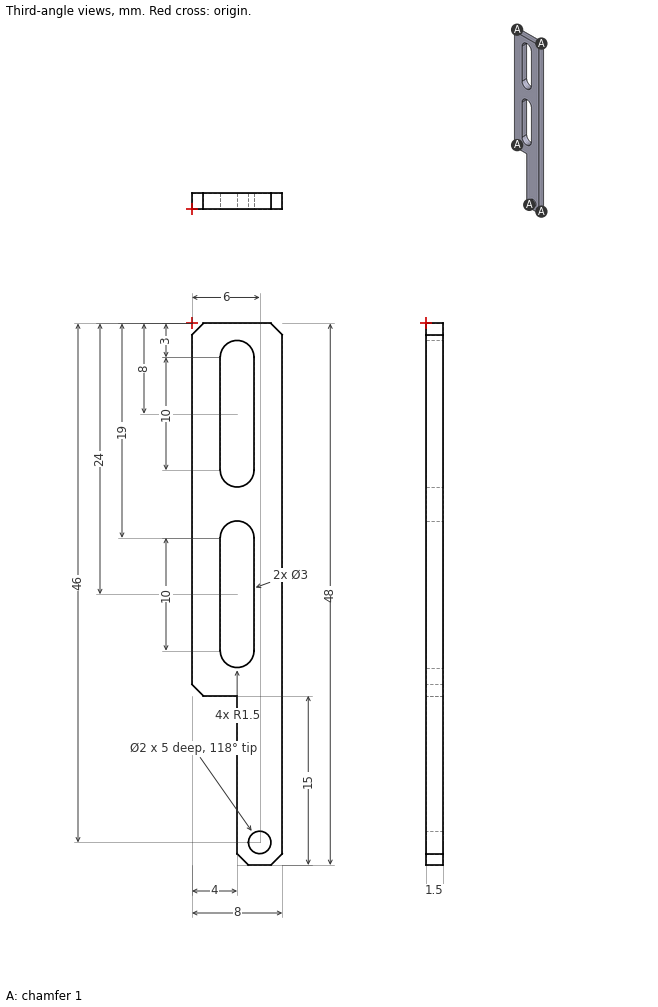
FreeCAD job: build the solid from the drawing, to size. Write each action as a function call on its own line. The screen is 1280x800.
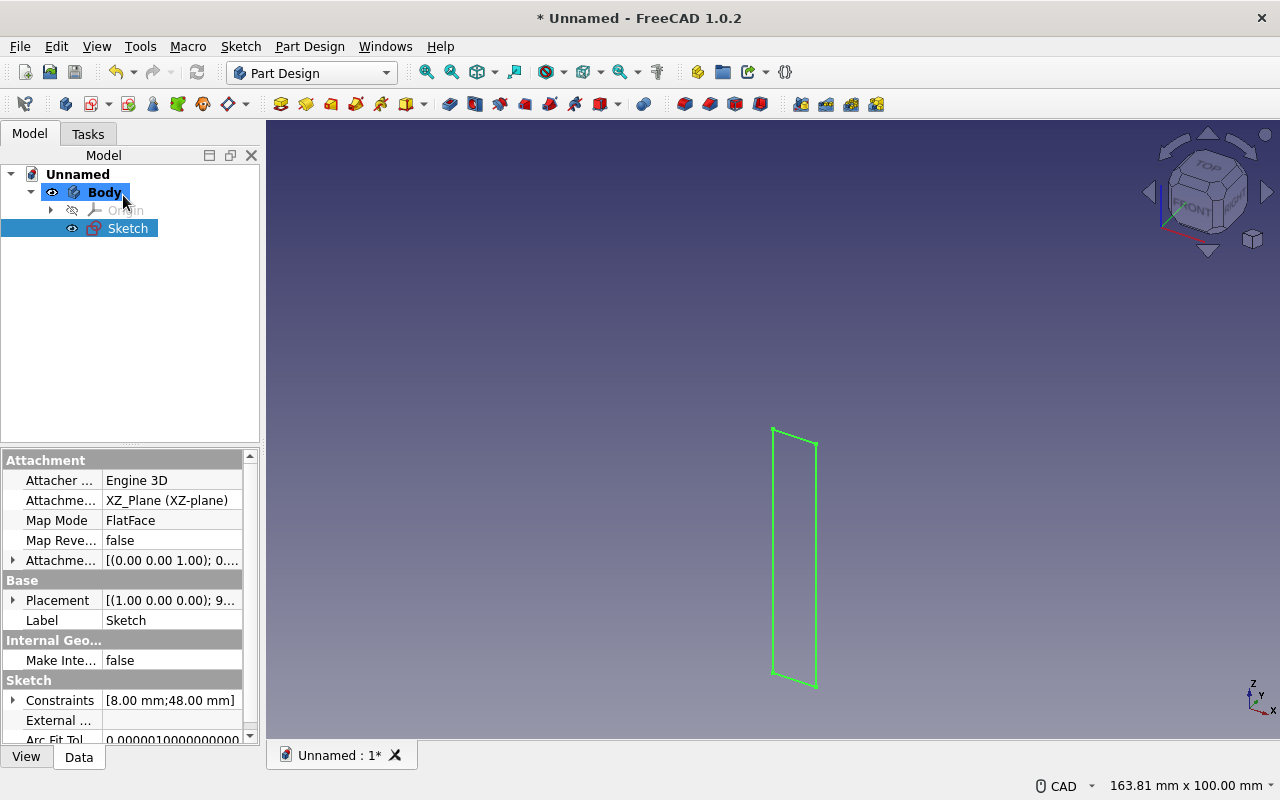
click(281, 104)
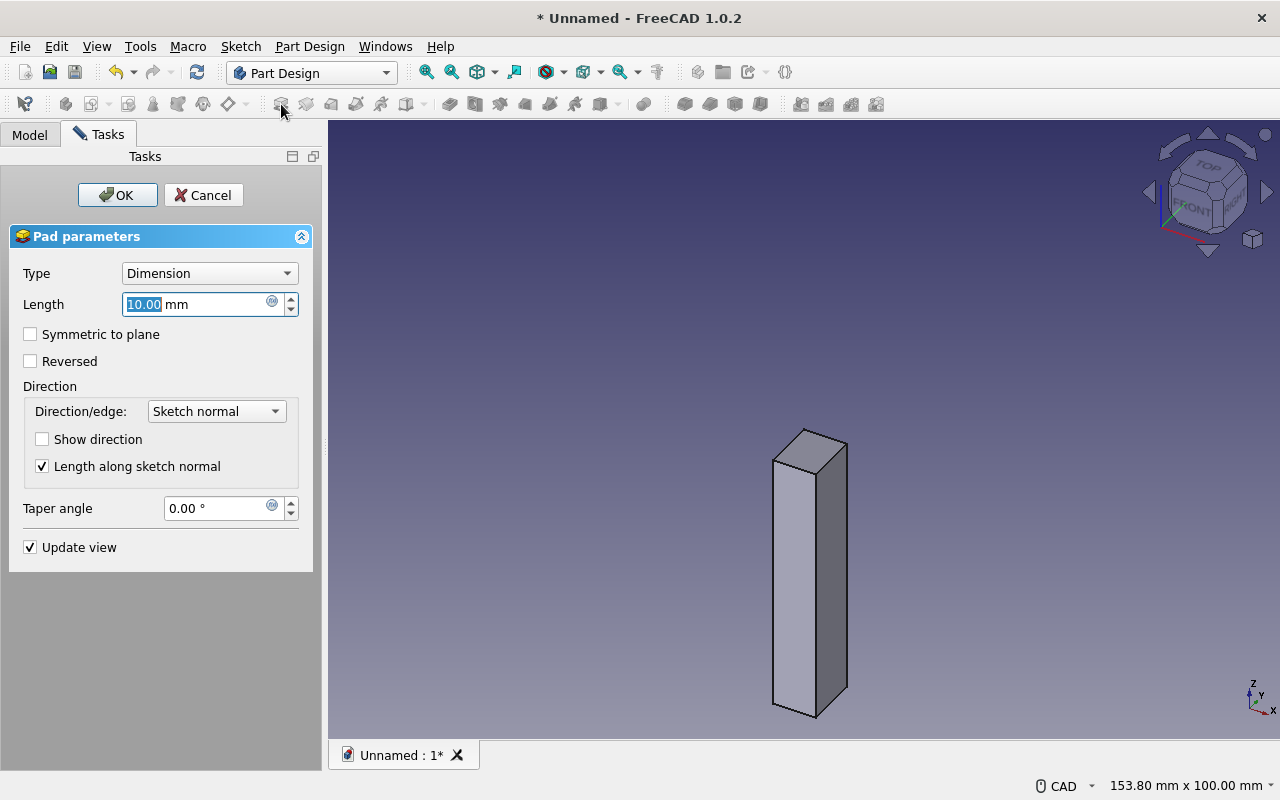
text(1.5)
key(Tab)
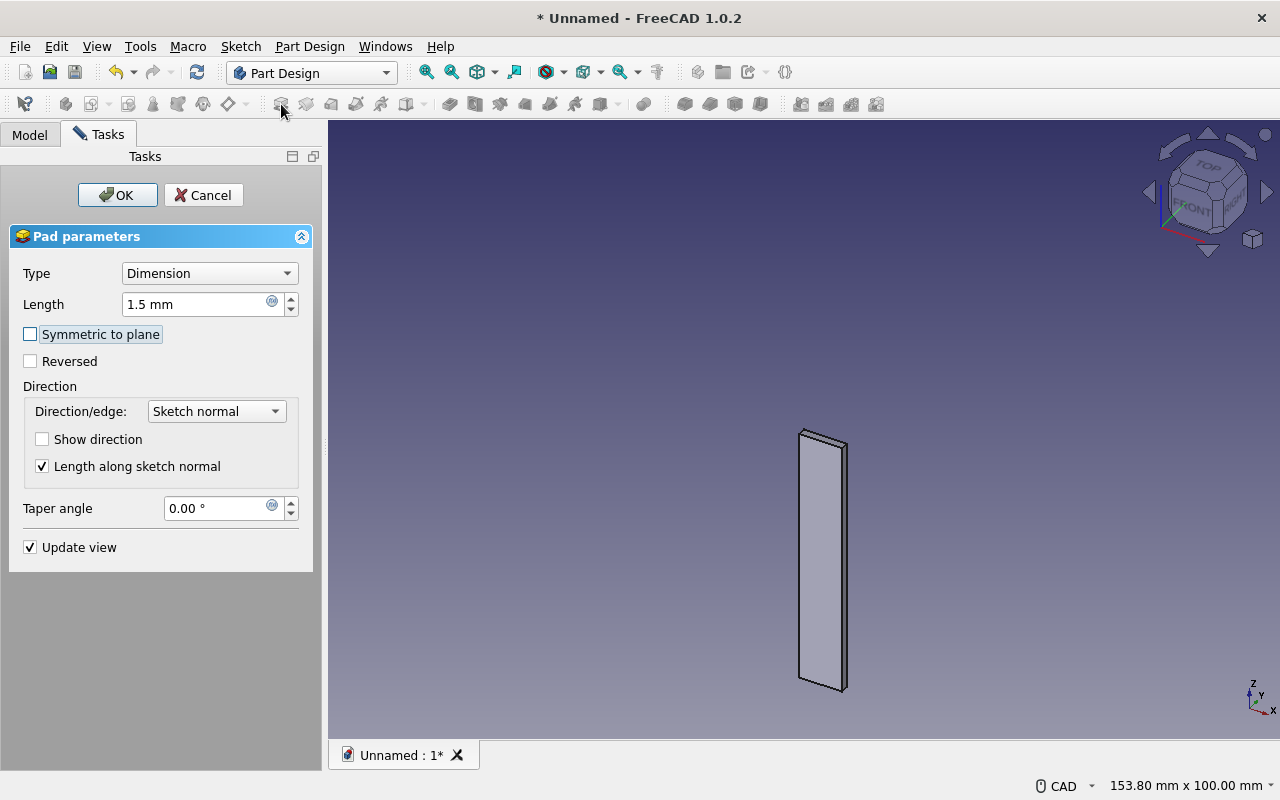
click(31, 361)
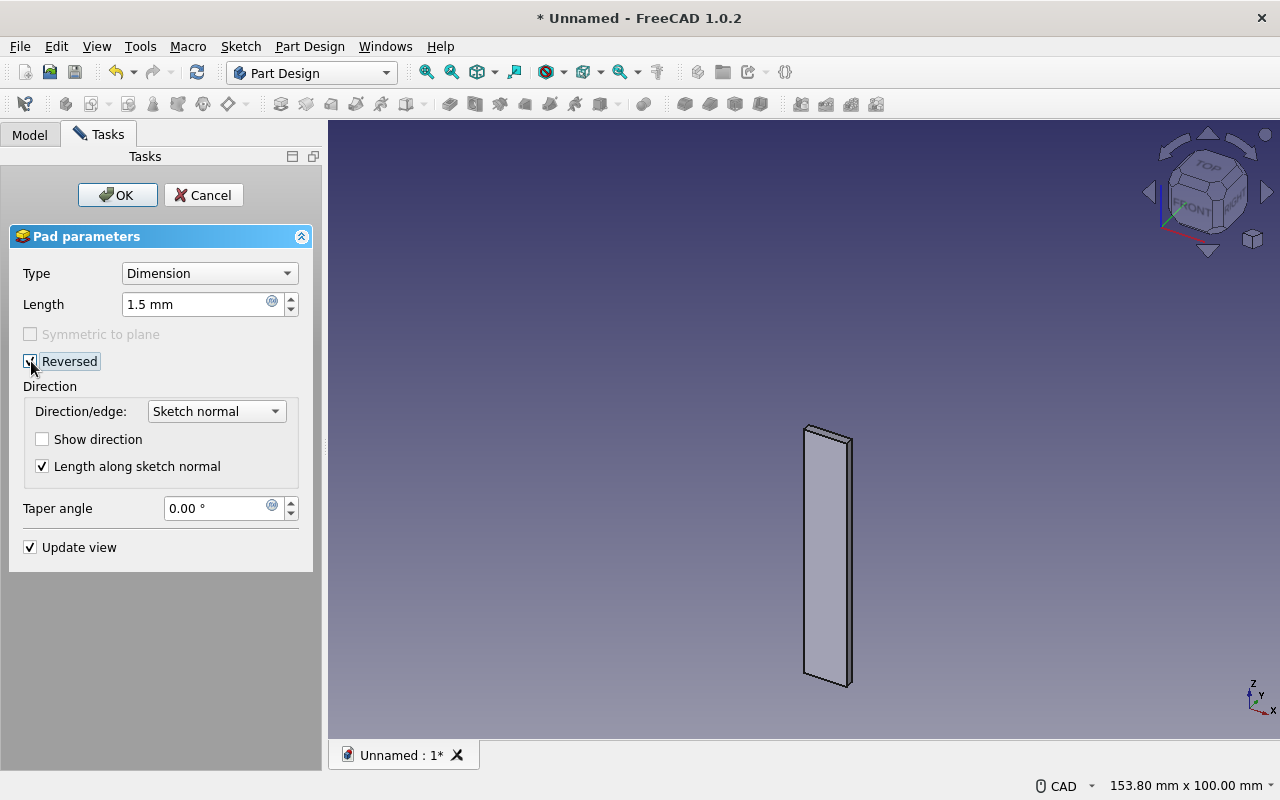
click(118, 195)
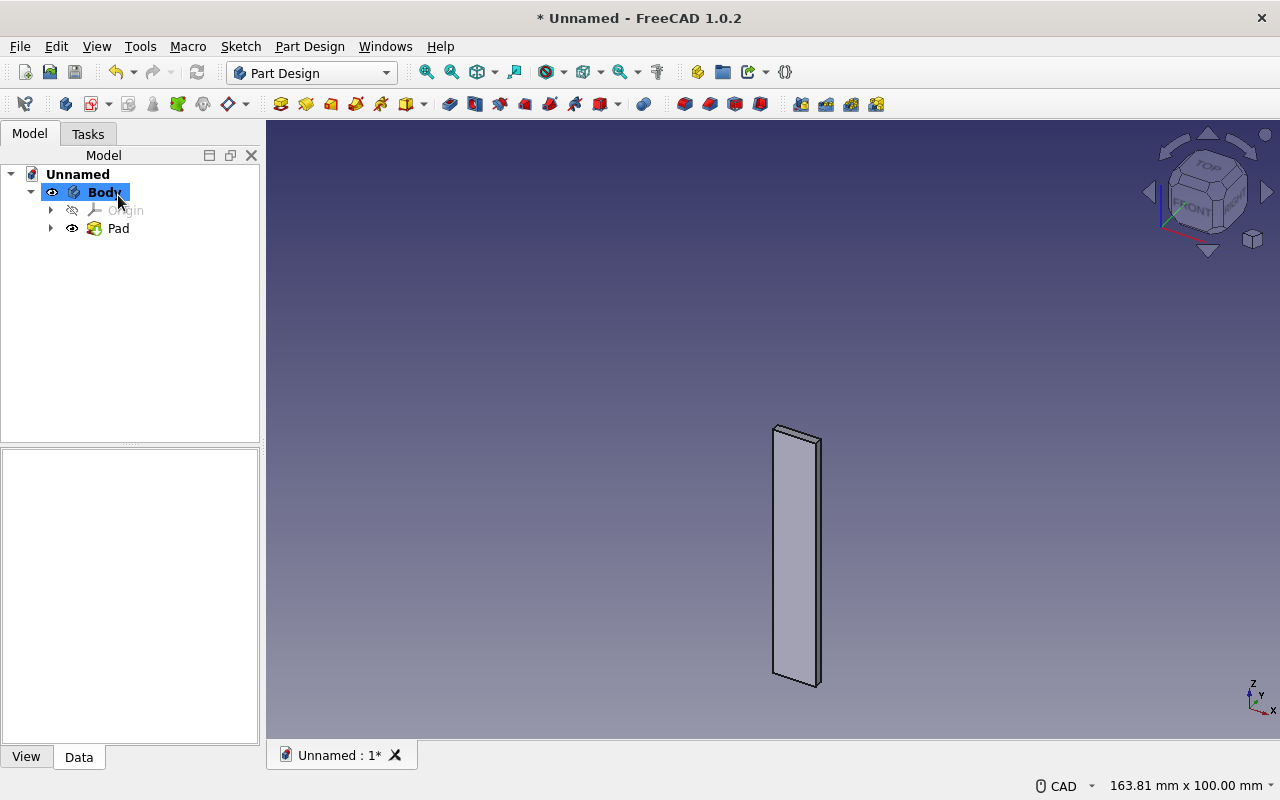
key(v)
key(f)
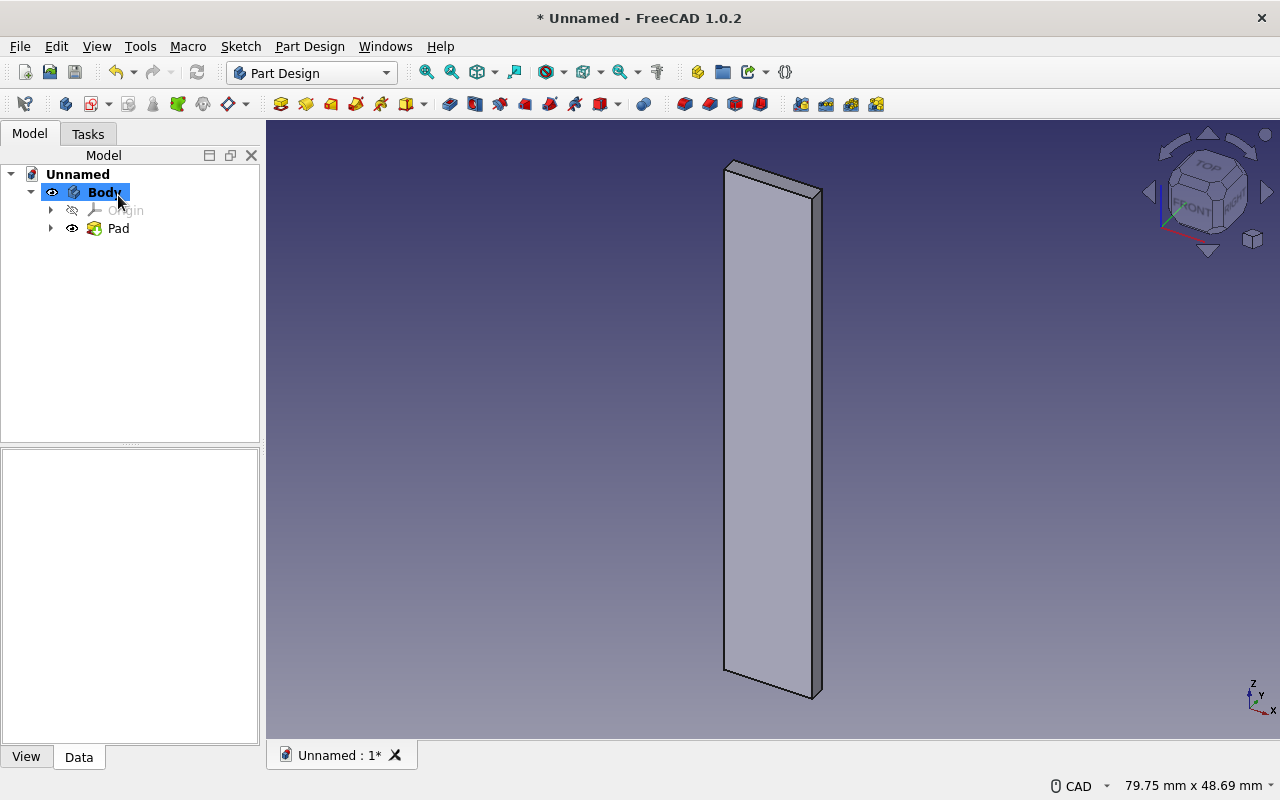
key(4)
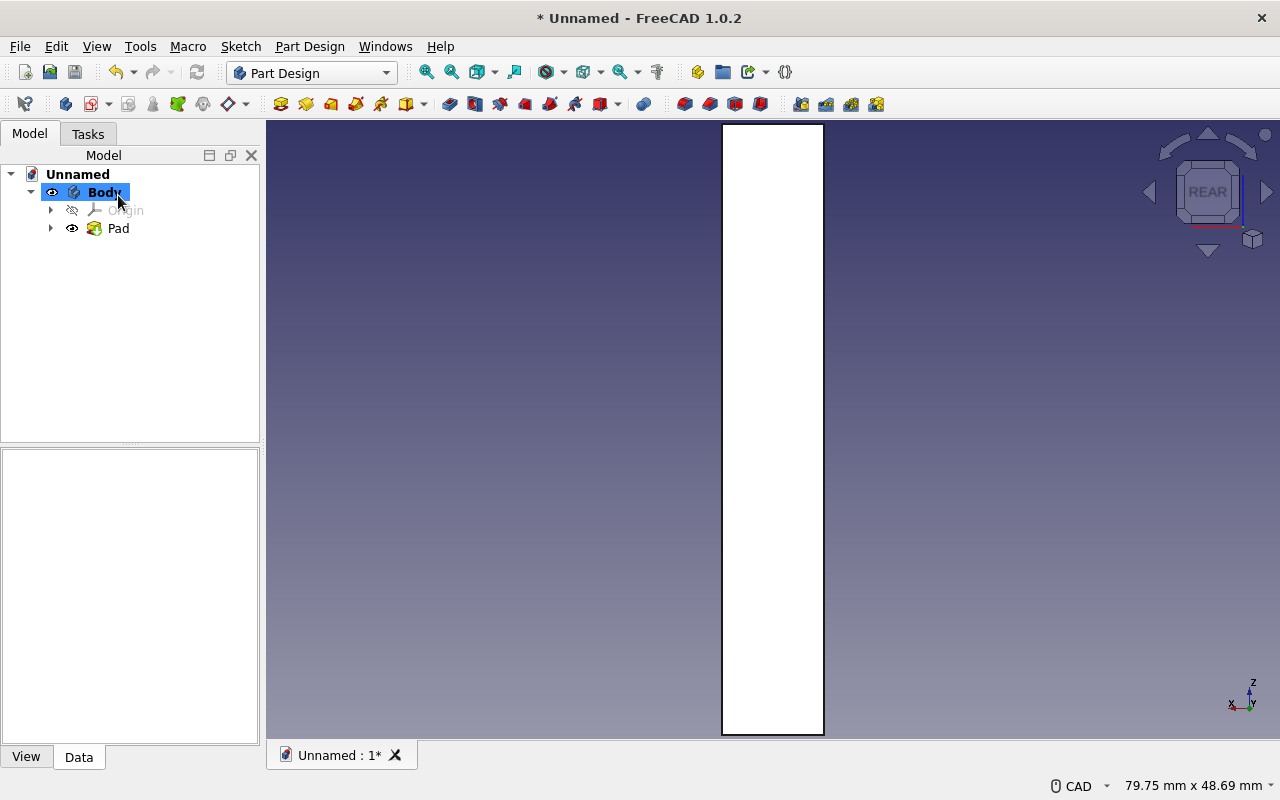
click(773, 254)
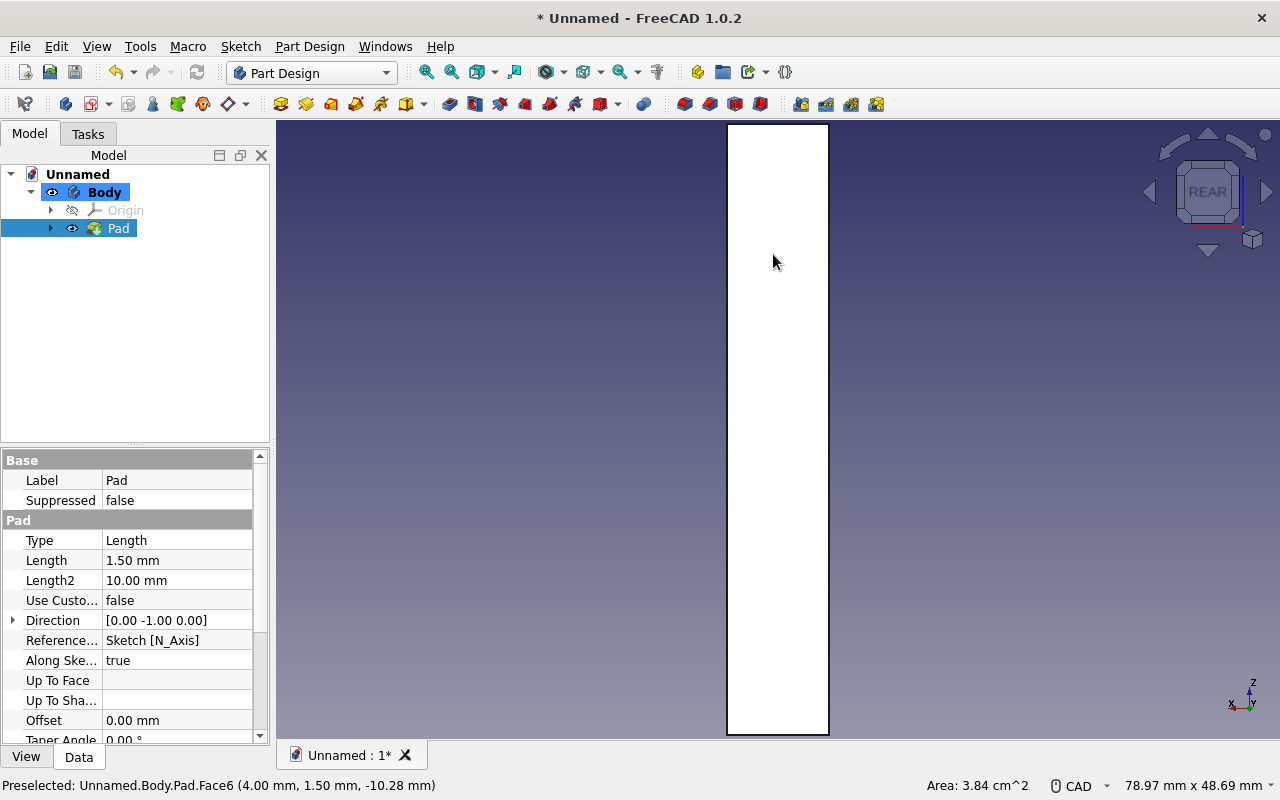
click(90, 104)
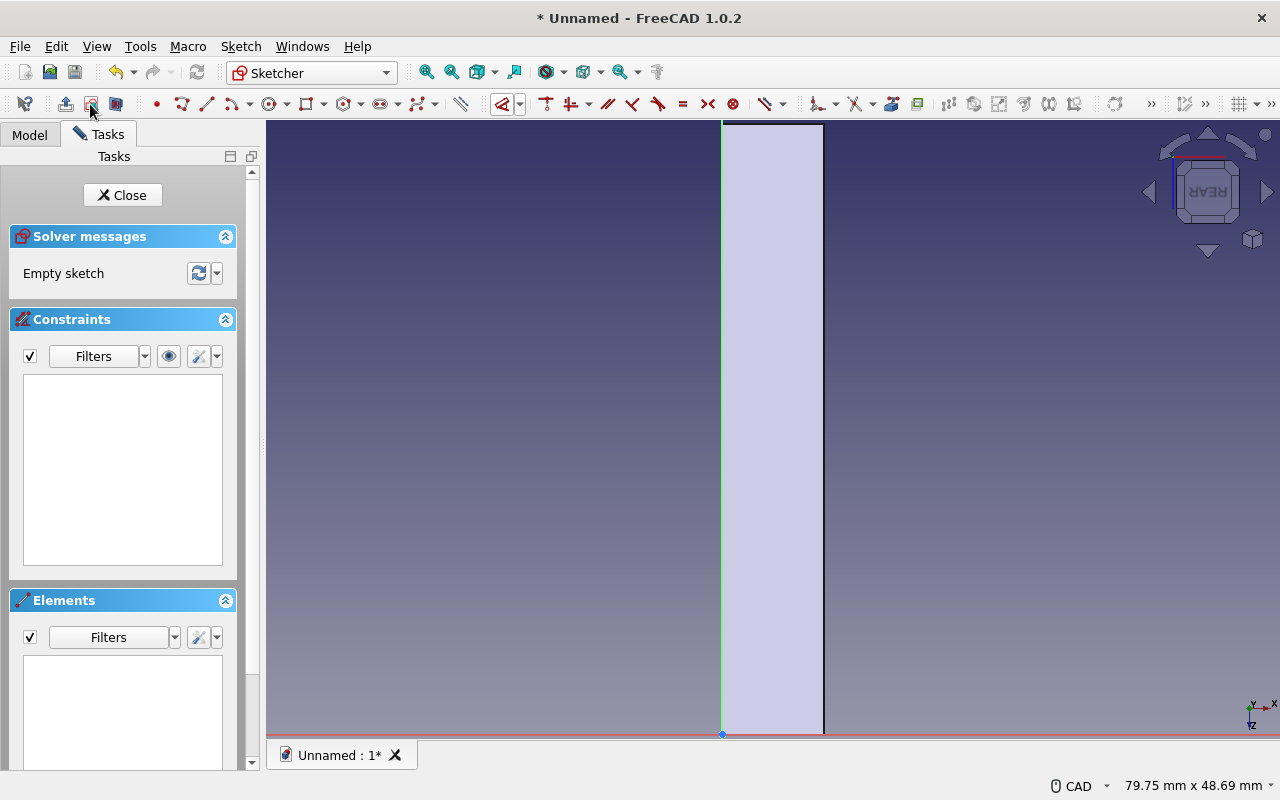
scroll(704, 430, down, 5)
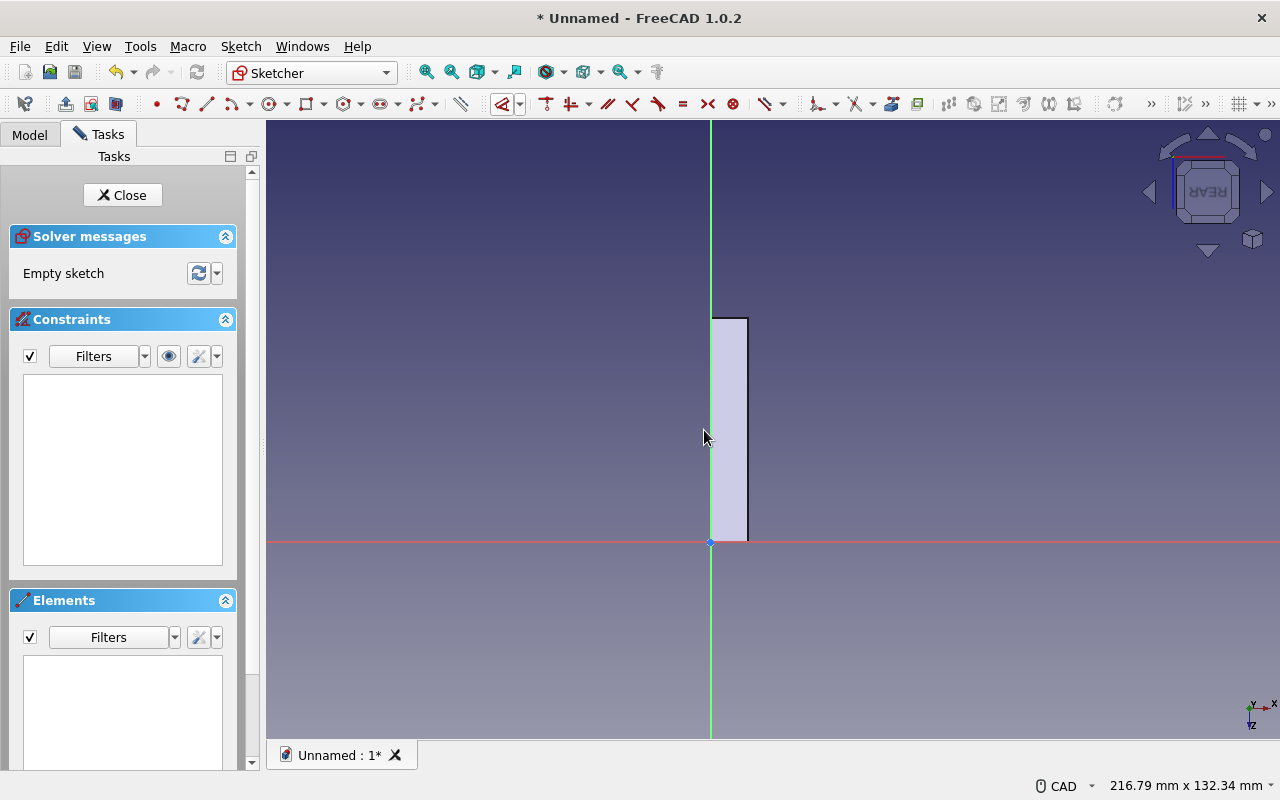
scroll(741, 322, up, 15)